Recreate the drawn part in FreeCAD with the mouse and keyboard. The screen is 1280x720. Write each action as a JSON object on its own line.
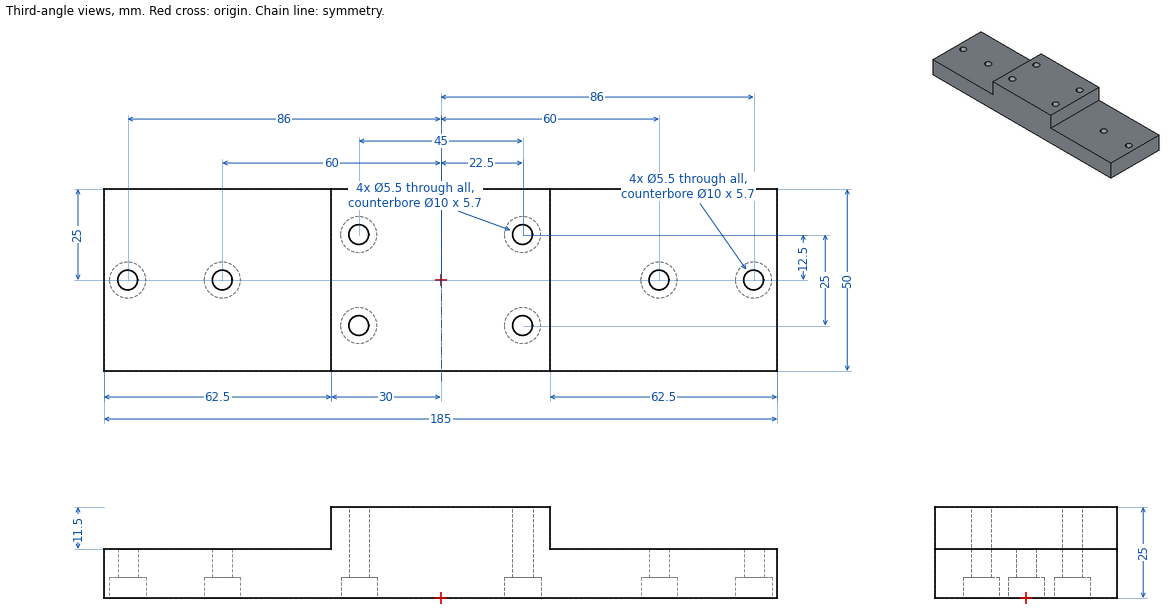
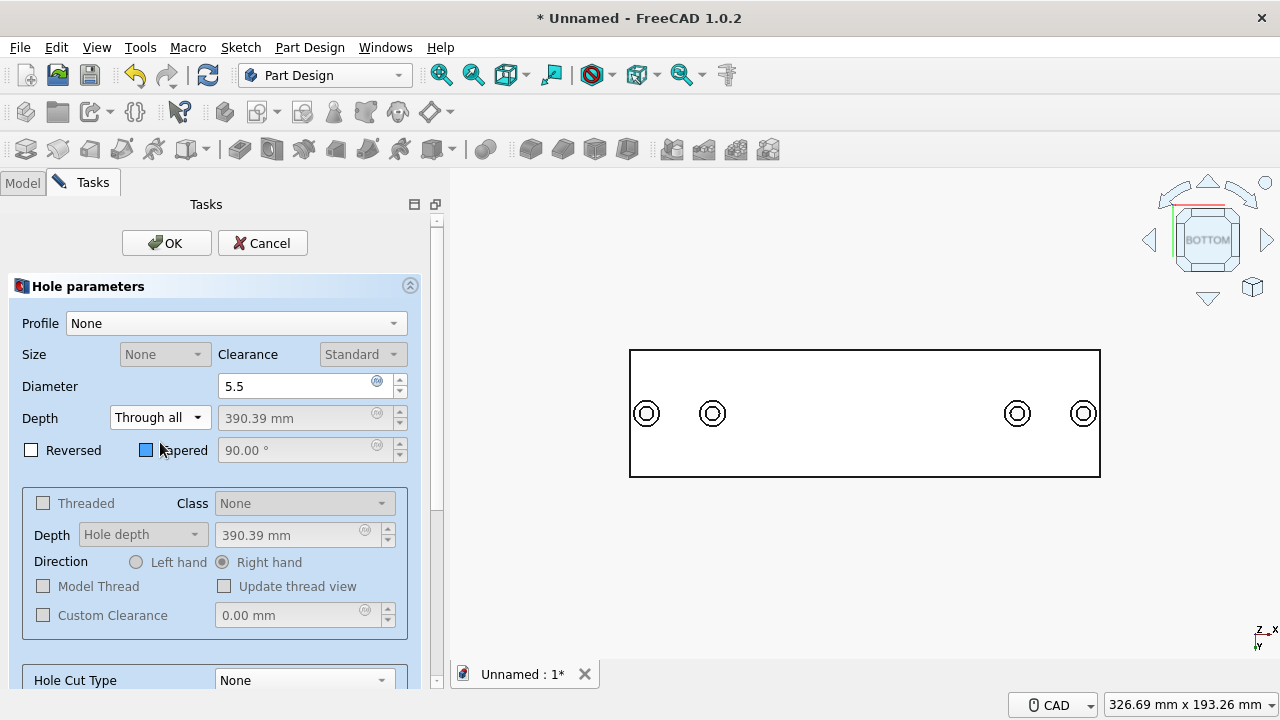
{"action": "left_click", "coordinate": [30, 450]}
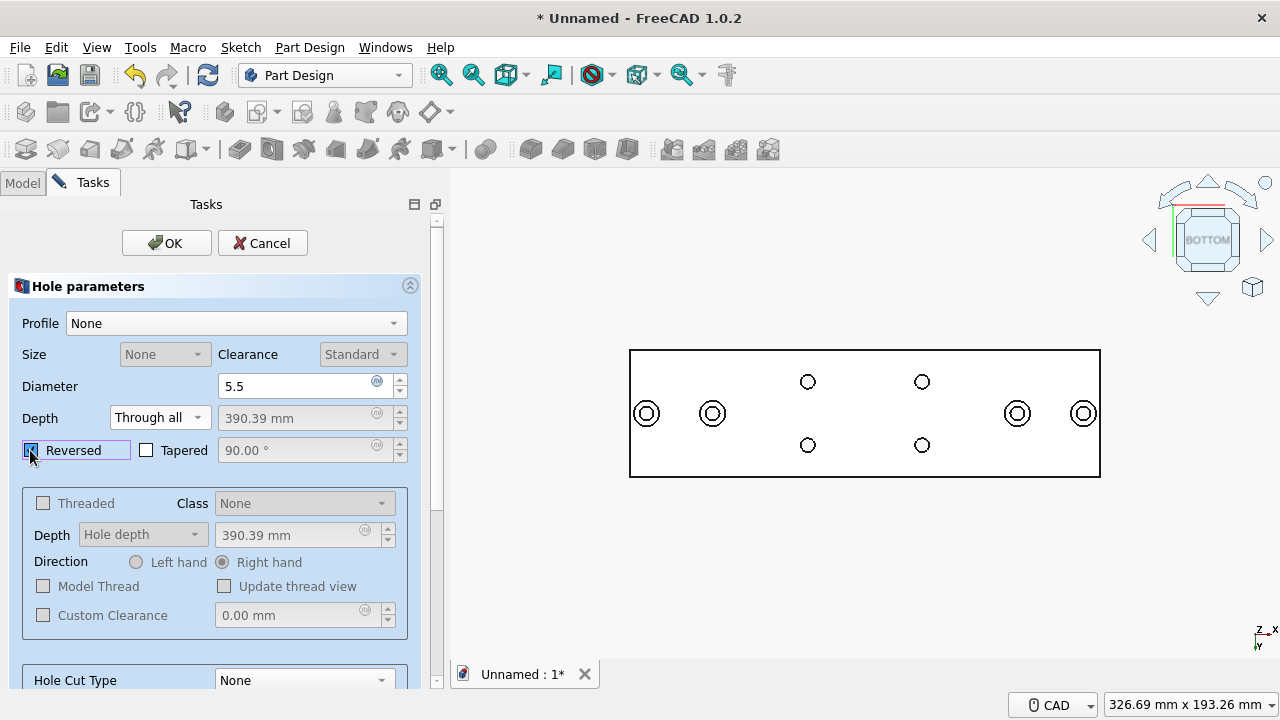
{"action": "scroll", "coordinate": [437, 451], "scroll_direction": "down", "scroll_amount": 2}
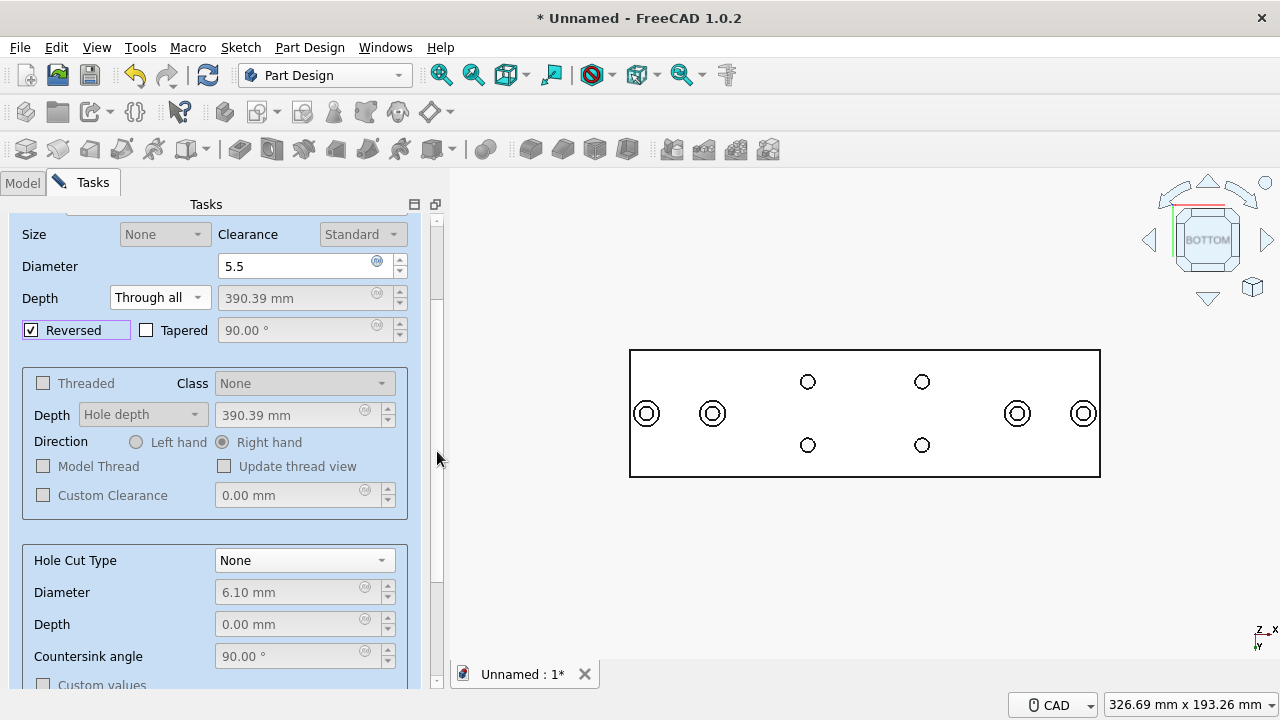
{"action": "left_click", "coordinate": [306, 560]}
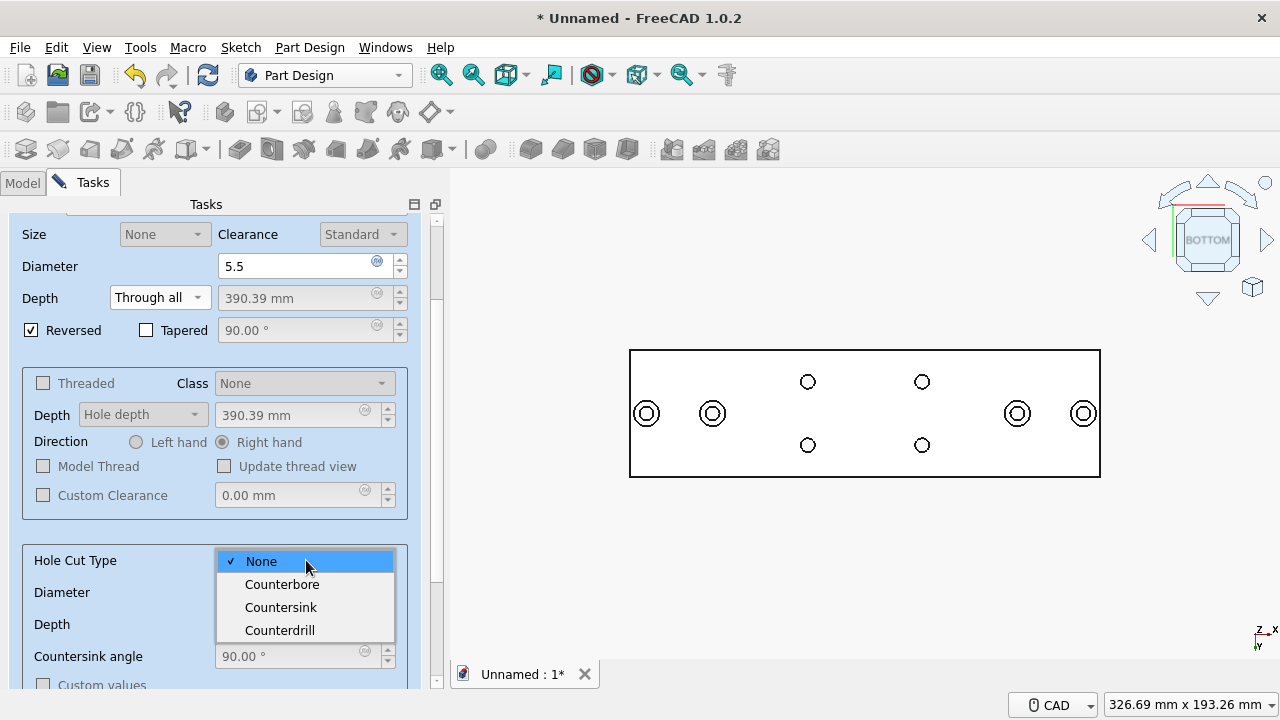
{"action": "left_click", "coordinate": [304, 584]}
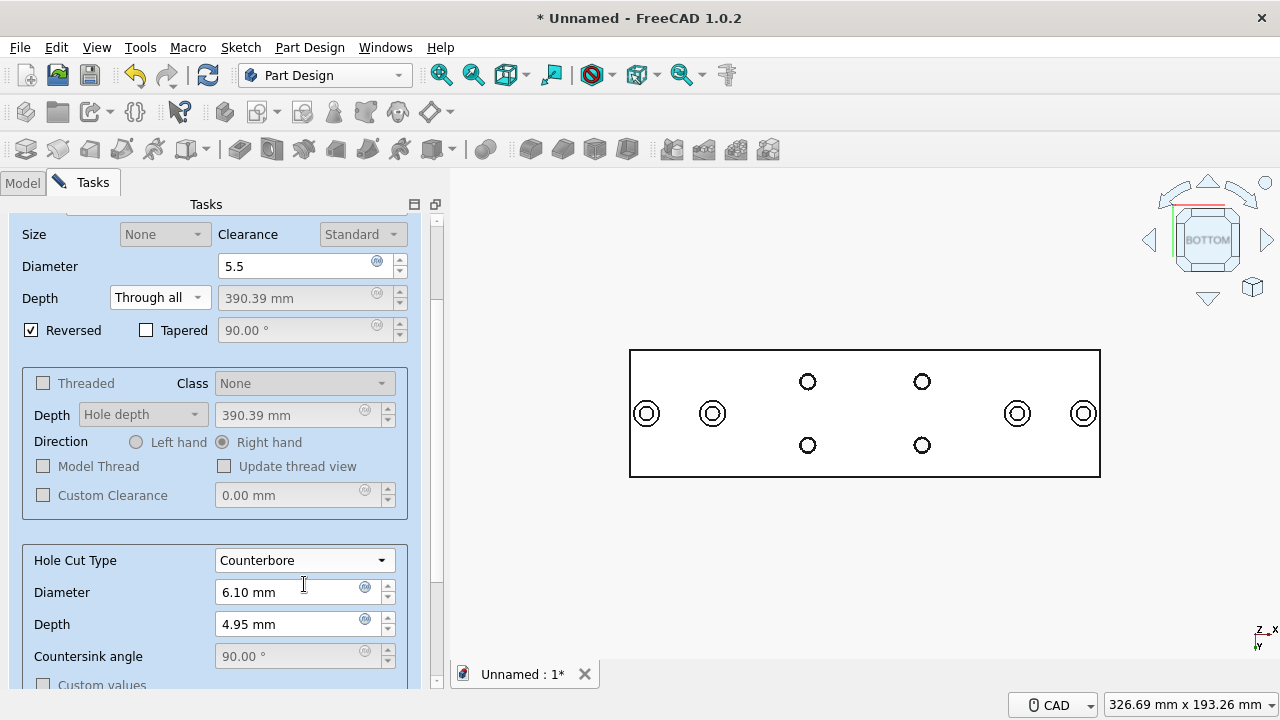
{"action": "triple_click", "coordinate": [298, 592]}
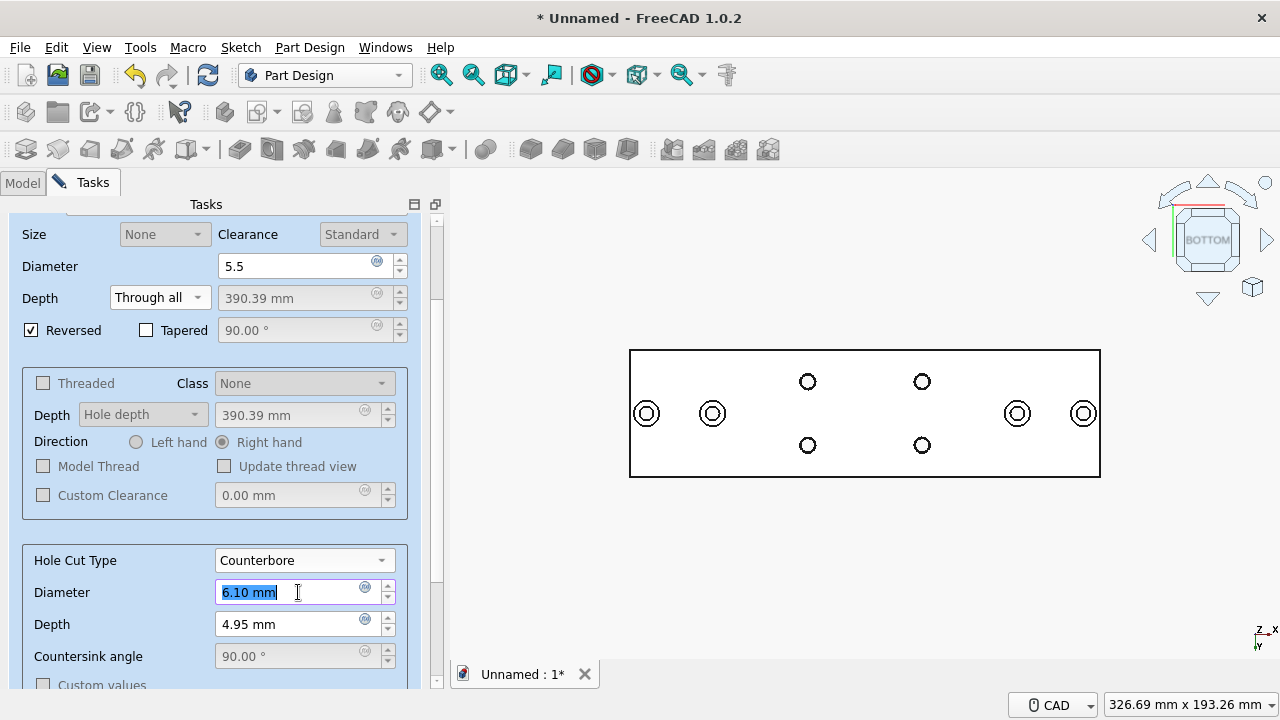
{"action": "type", "text": "10"}
{"action": "key", "text": "Tab"}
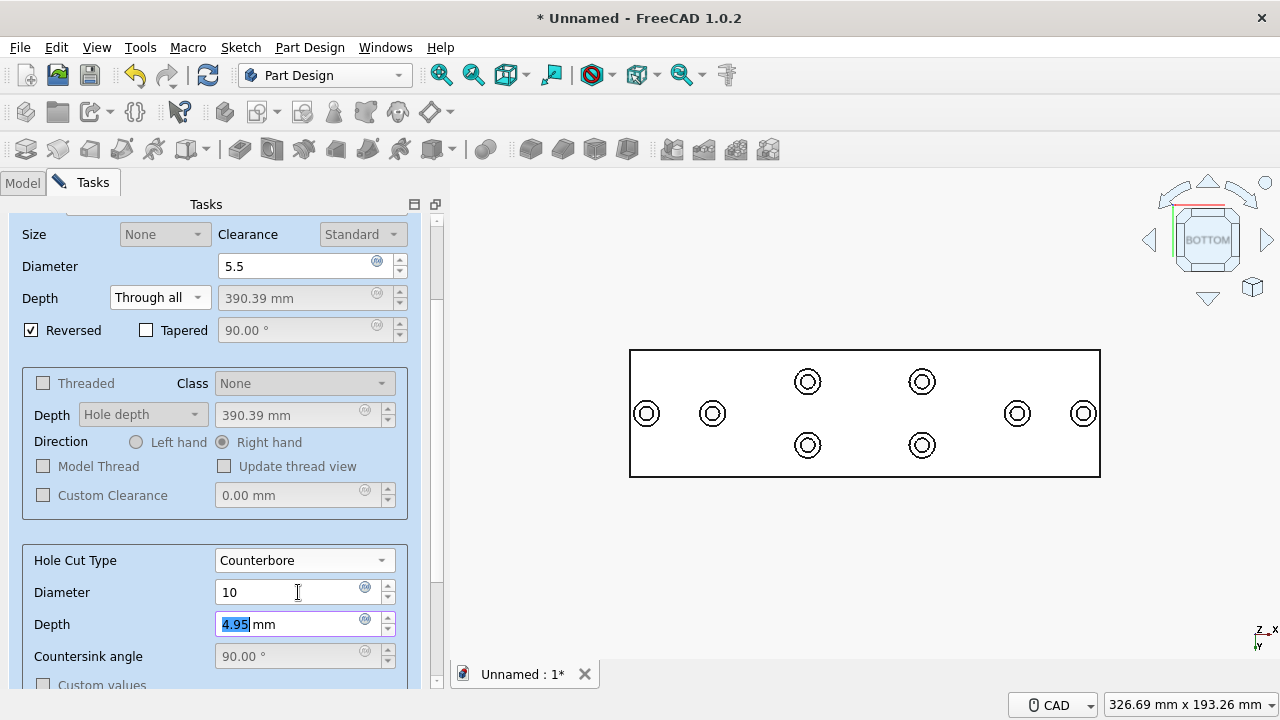
{"action": "type", "text": "5.7"}
{"action": "key", "text": "Tab"}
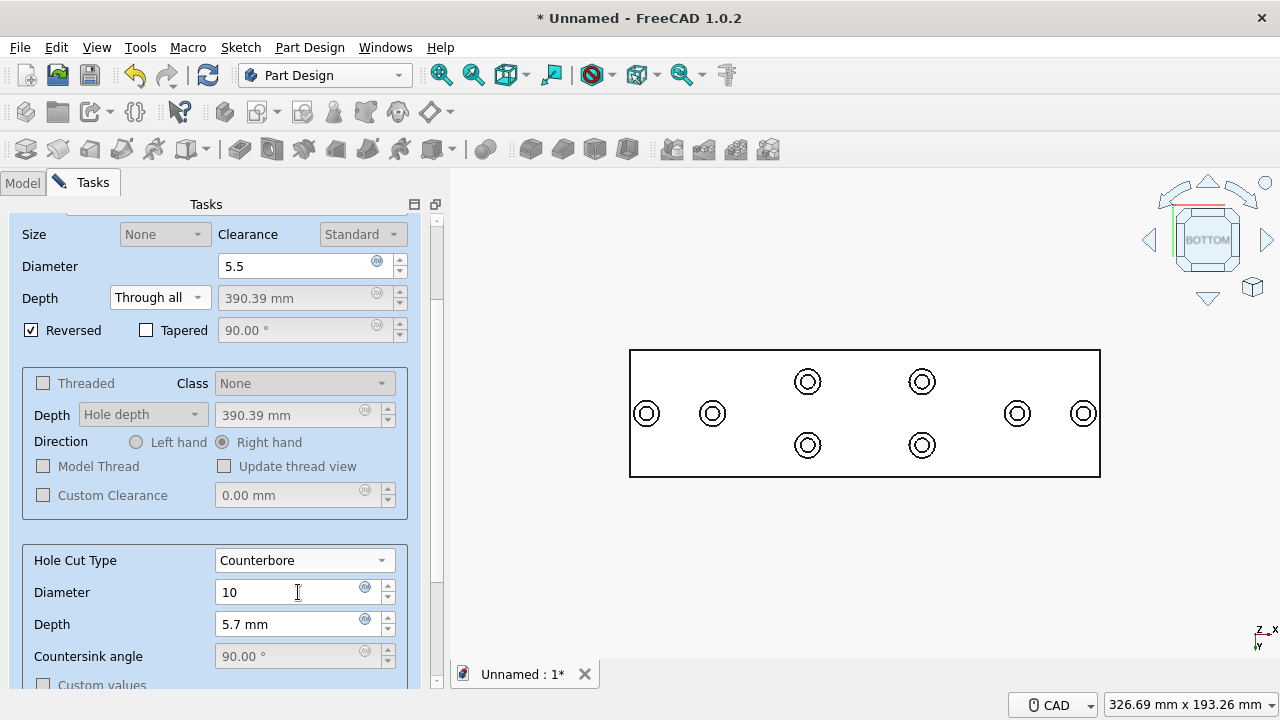
{"action": "scroll", "coordinate": [437, 451], "scroll_direction": "up", "scroll_amount": 3}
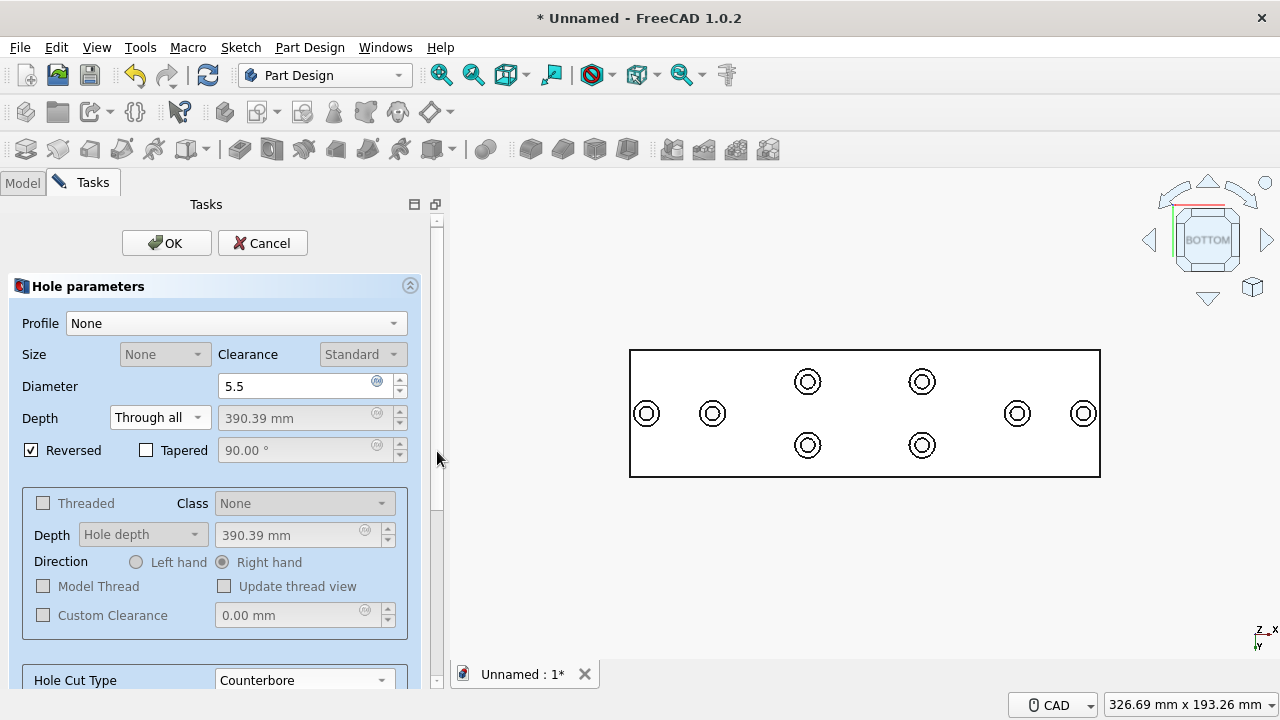
{"action": "left_click", "coordinate": [167, 243]}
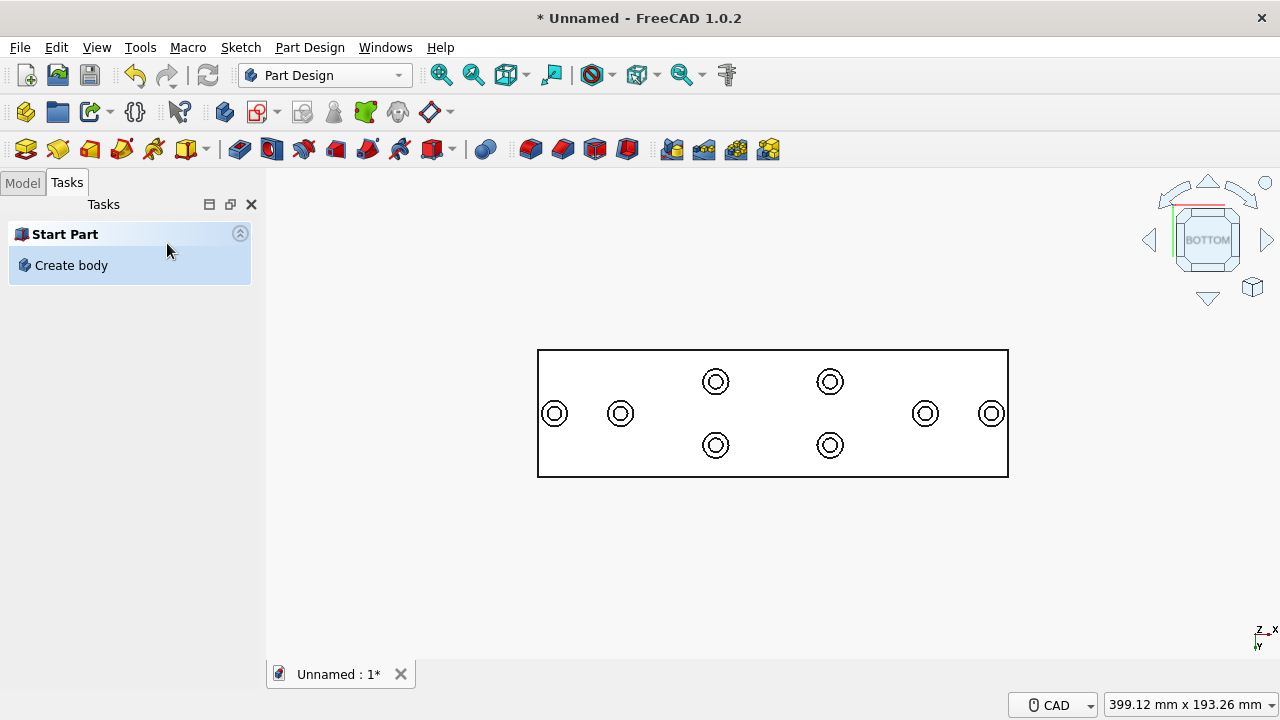
{"action": "key", "text": "0"}